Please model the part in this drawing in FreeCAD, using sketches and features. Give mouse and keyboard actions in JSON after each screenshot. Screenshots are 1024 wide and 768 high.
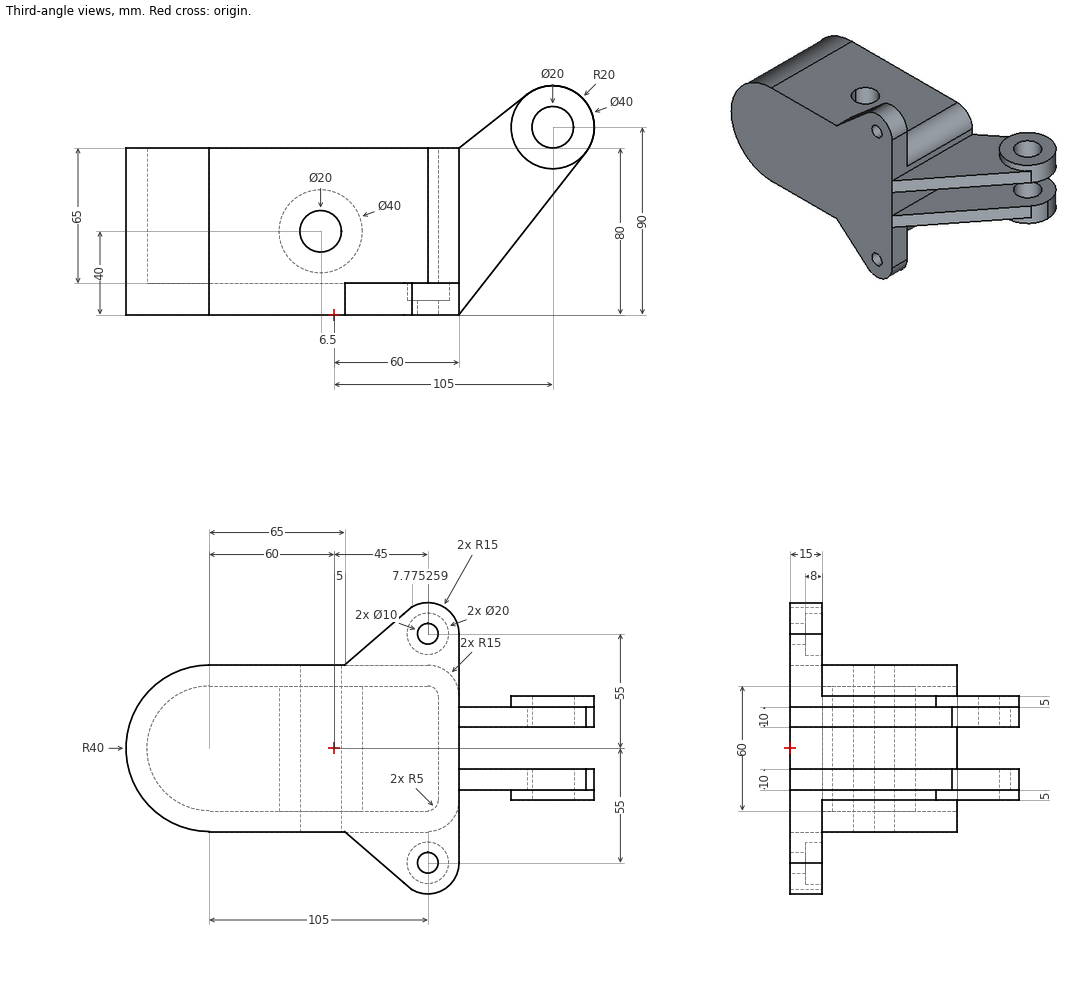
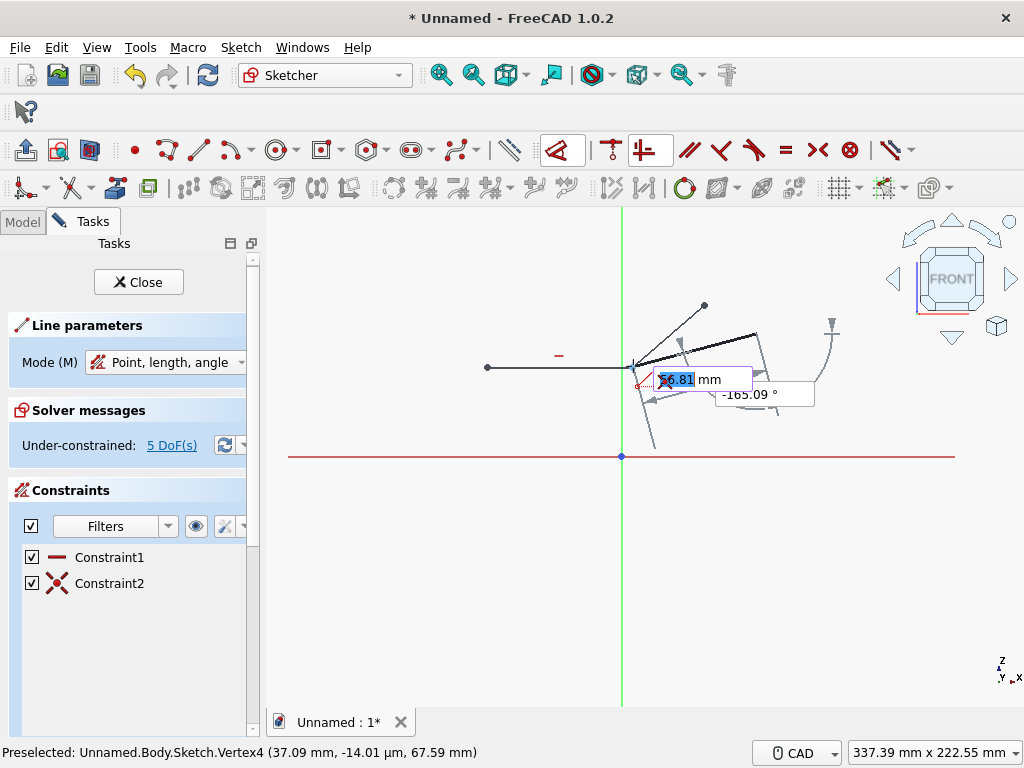
{"action": "left_click", "coordinate": [756, 581]}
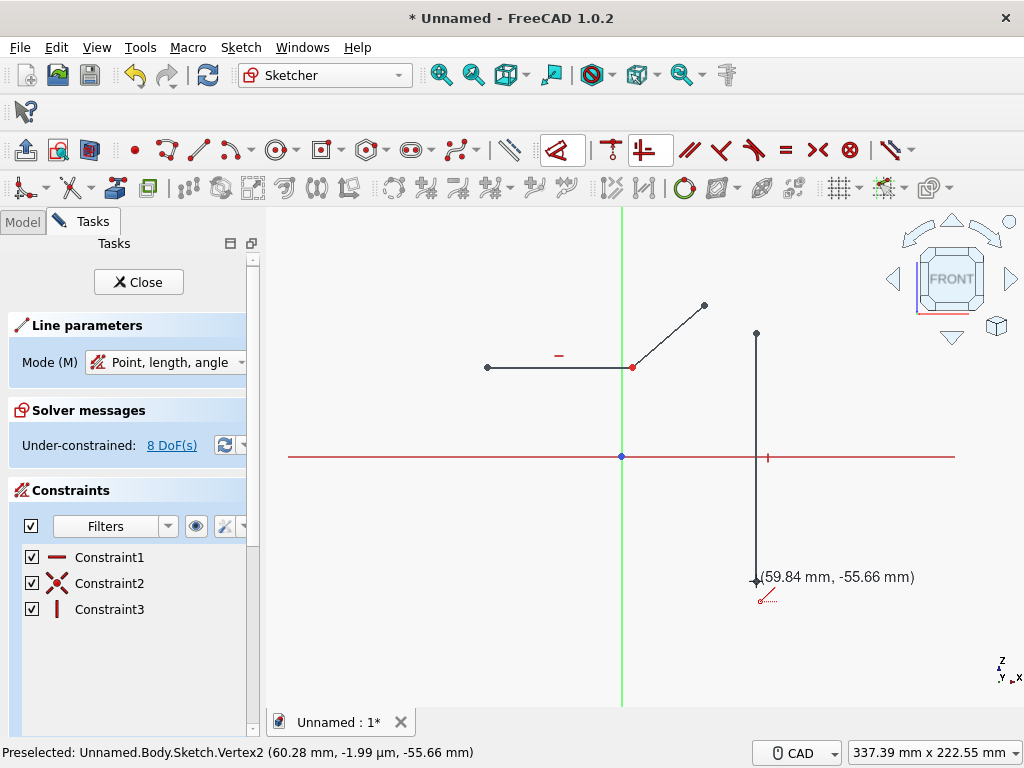
{"action": "left_click", "coordinate": [168, 150]}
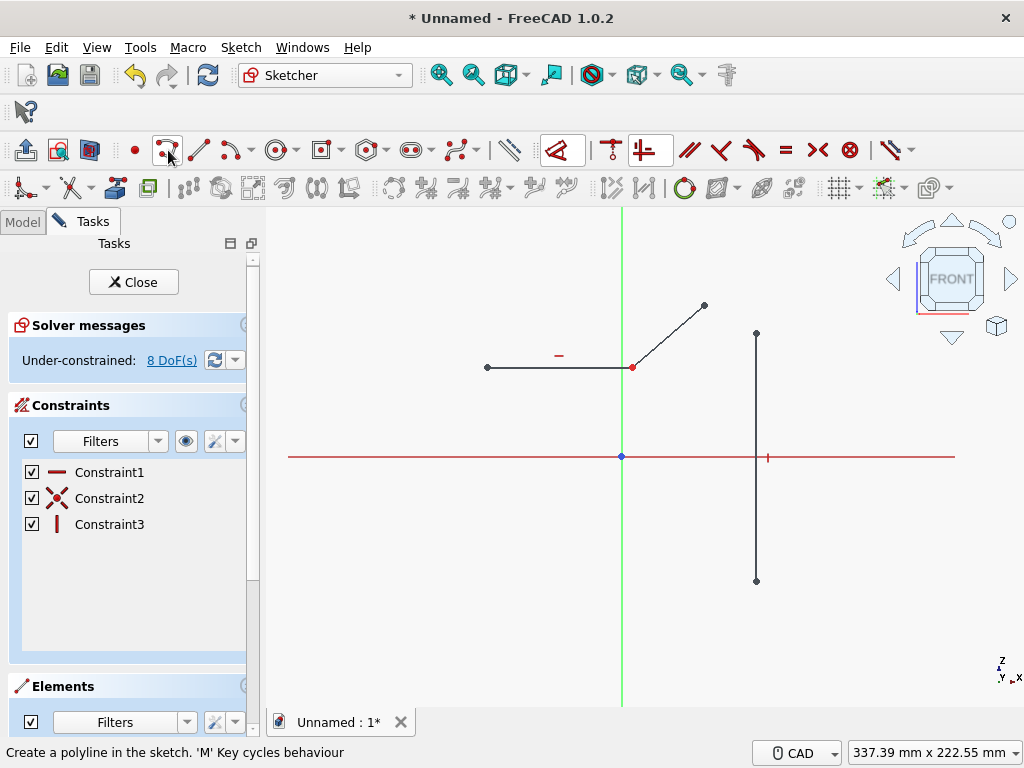
{"action": "left_click", "coordinate": [705, 609]}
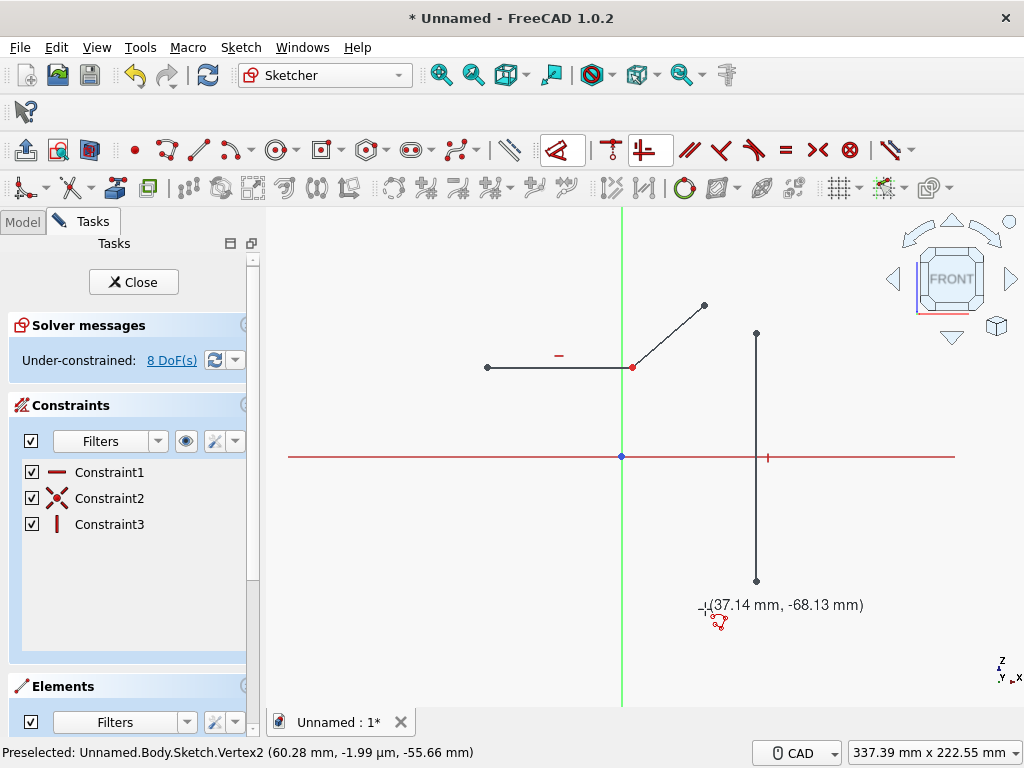
{"action": "scroll", "coordinate": [633, 547], "scroll_direction": "up", "scroll_amount": 2}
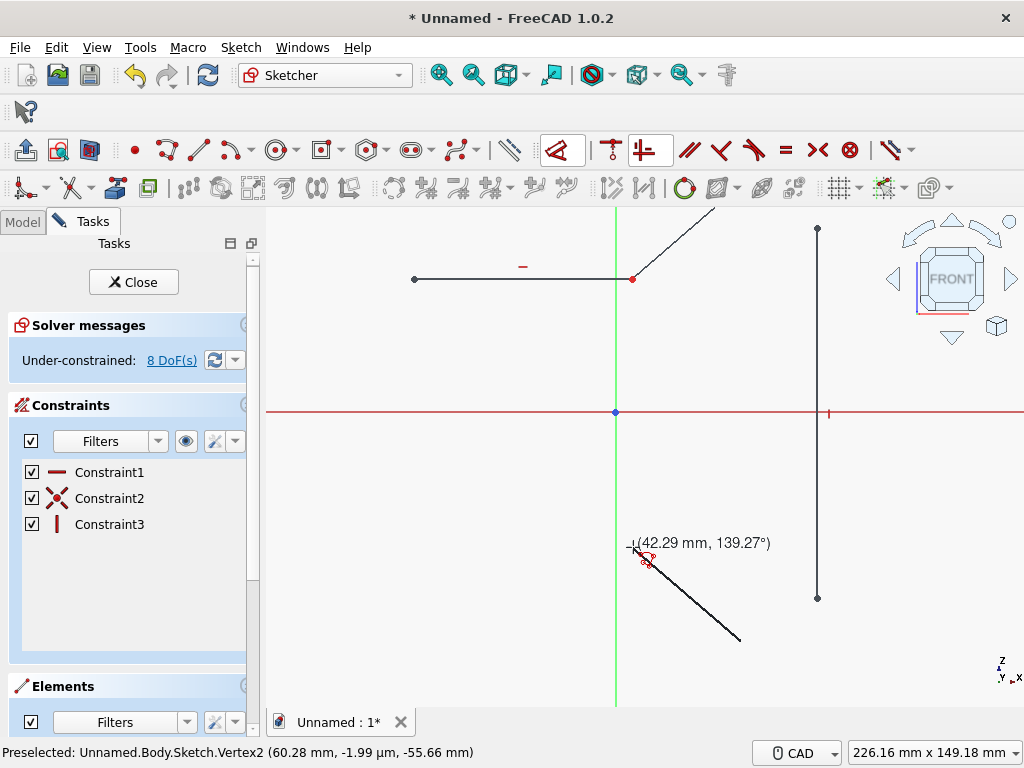
{"action": "left_click", "coordinate": [632, 546]}
{"action": "left_click", "coordinate": [415, 546]}
{"action": "right_click", "coordinate": [415, 546]}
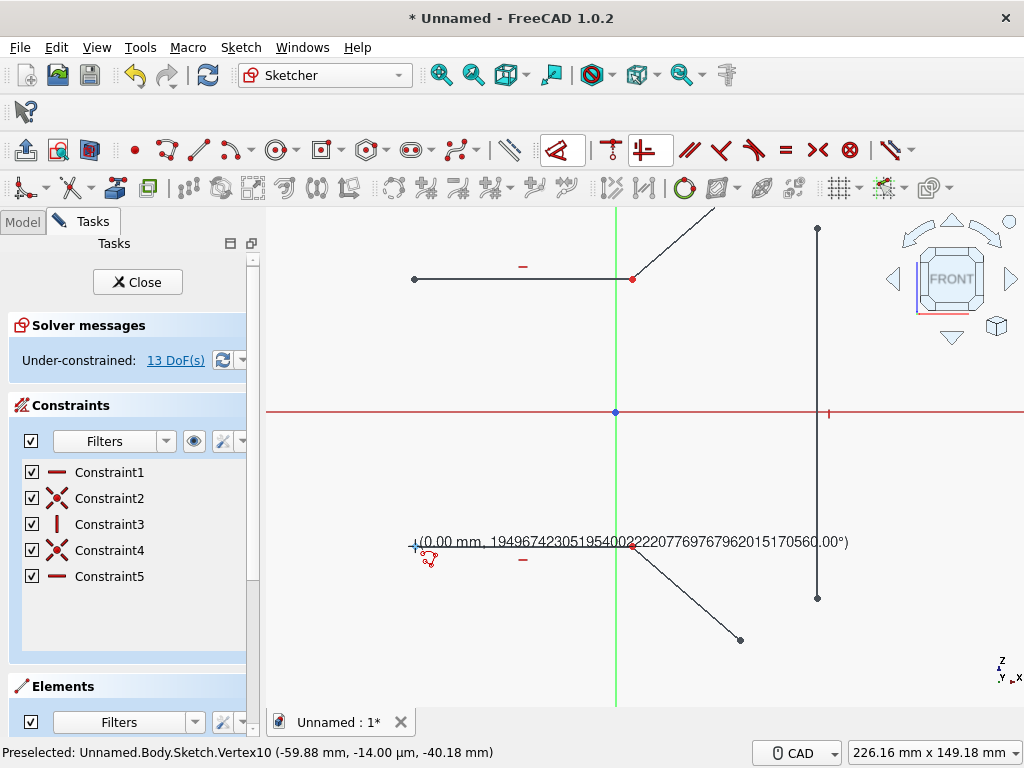
{"action": "left_click", "coordinate": [254, 150]}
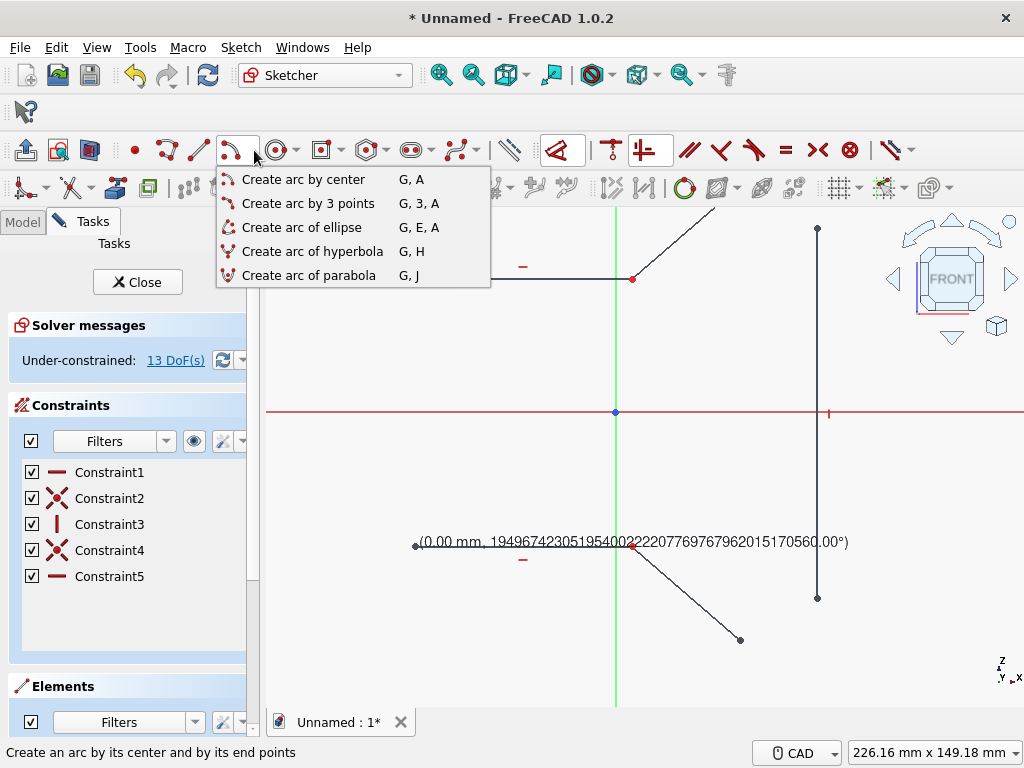
{"action": "left_click", "coordinate": [354, 203]}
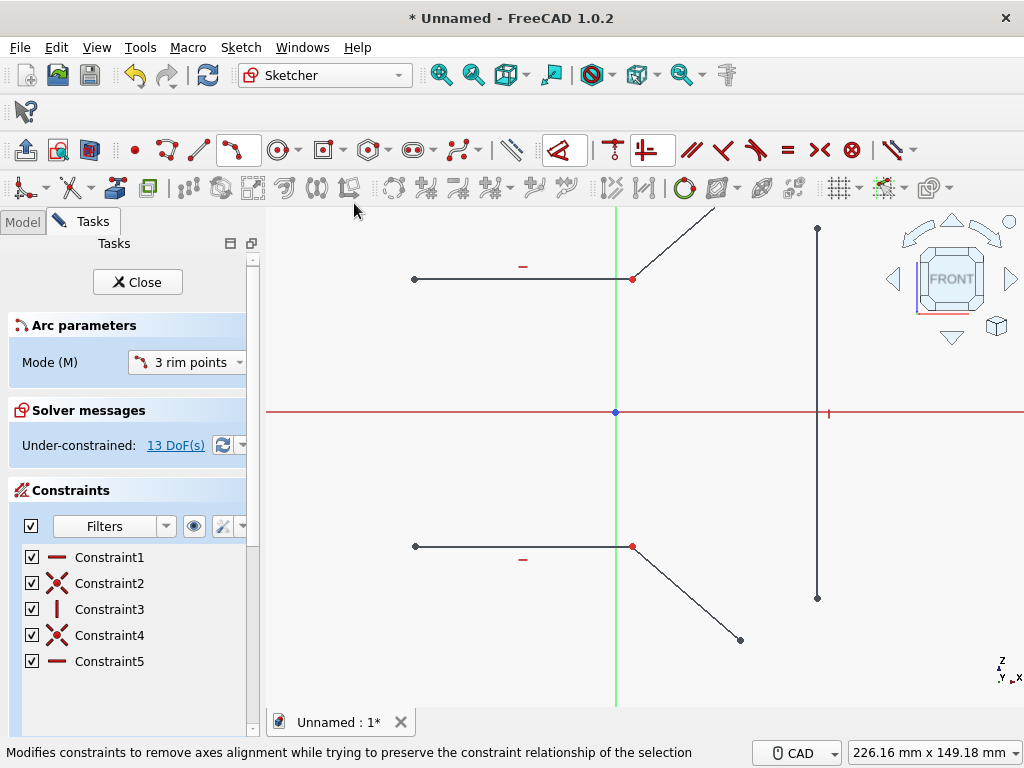
{"action": "scroll", "coordinate": [633, 548], "scroll_direction": "down", "scroll_amount": 2}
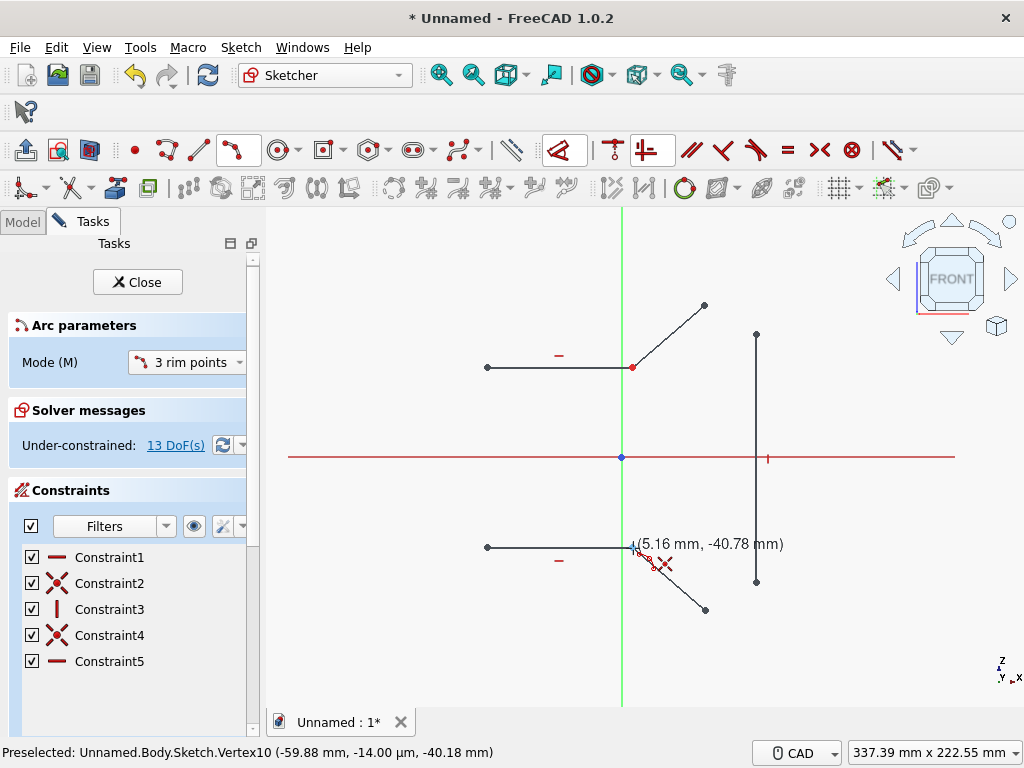
{"action": "left_click", "coordinate": [705, 305]}
{"action": "left_click", "coordinate": [756, 334]}
{"action": "left_click", "coordinate": [739, 304]}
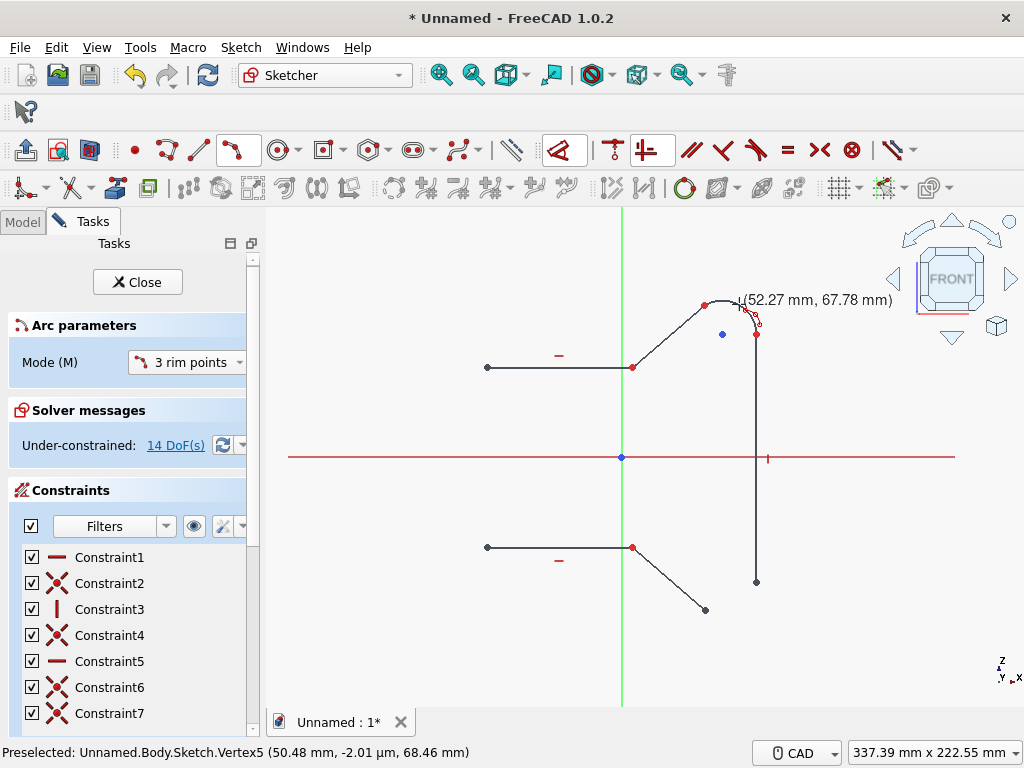
{"action": "left_click", "coordinate": [756, 582]}
{"action": "left_click", "coordinate": [705, 610]}
{"action": "left_click", "coordinate": [739, 610]}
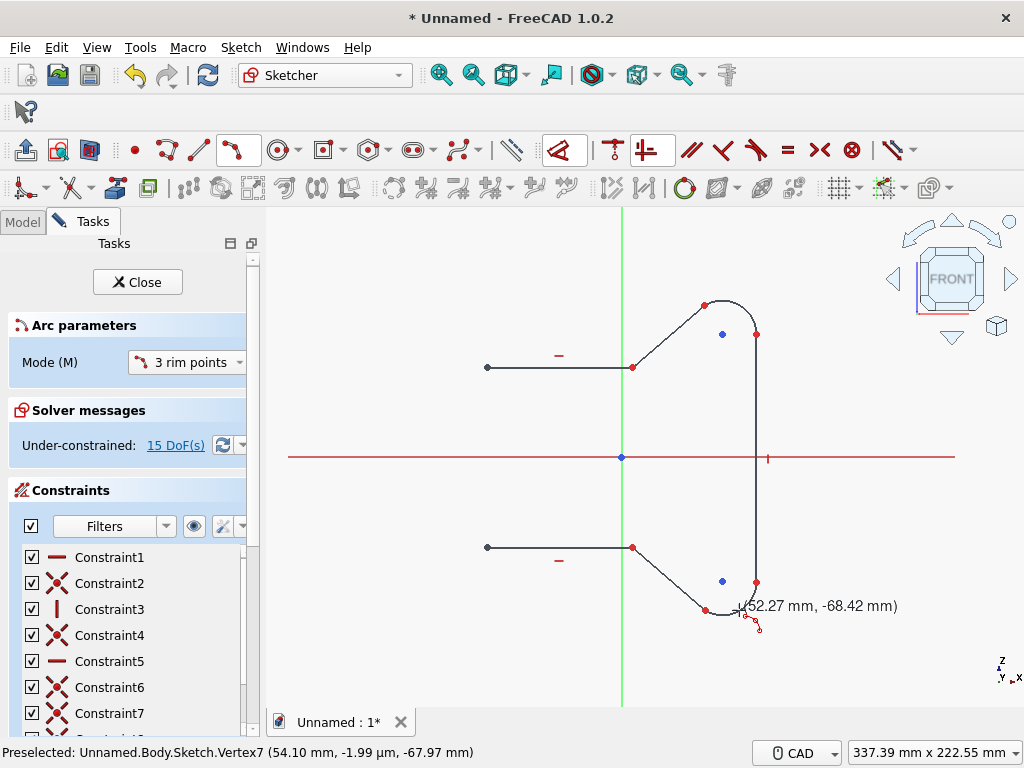
{"action": "left_click", "coordinate": [487, 548]}
{"action": "left_click", "coordinate": [487, 368]}
{"action": "left_click", "coordinate": [401, 430]}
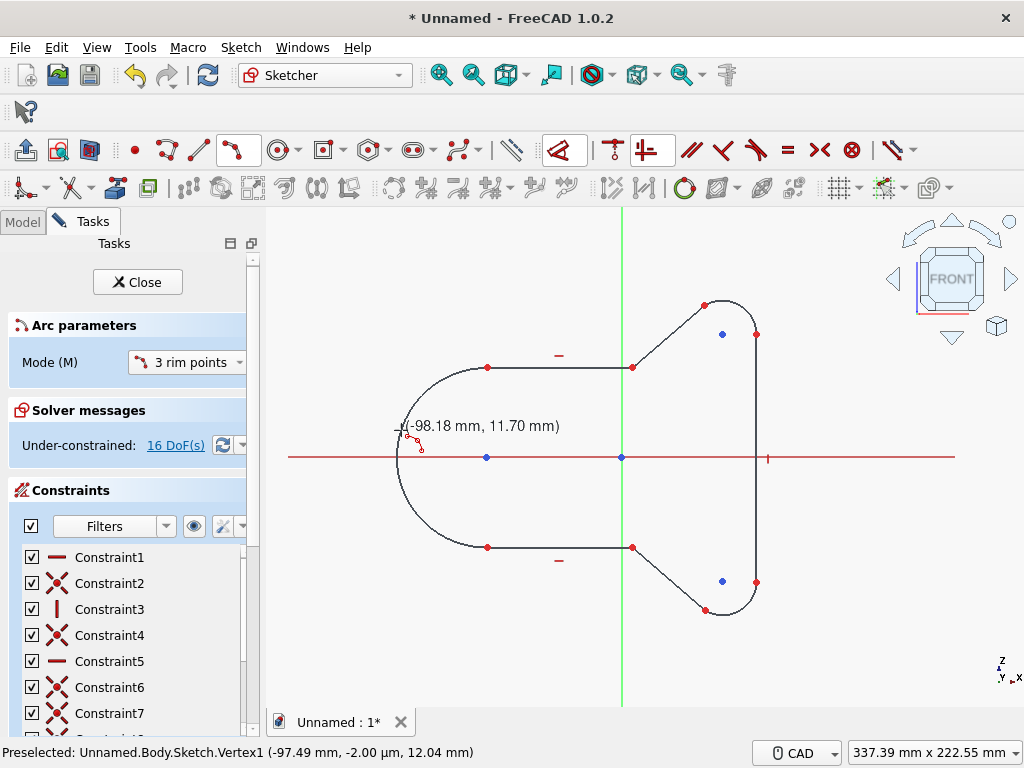
{"action": "left_click", "coordinate": [278, 150]}